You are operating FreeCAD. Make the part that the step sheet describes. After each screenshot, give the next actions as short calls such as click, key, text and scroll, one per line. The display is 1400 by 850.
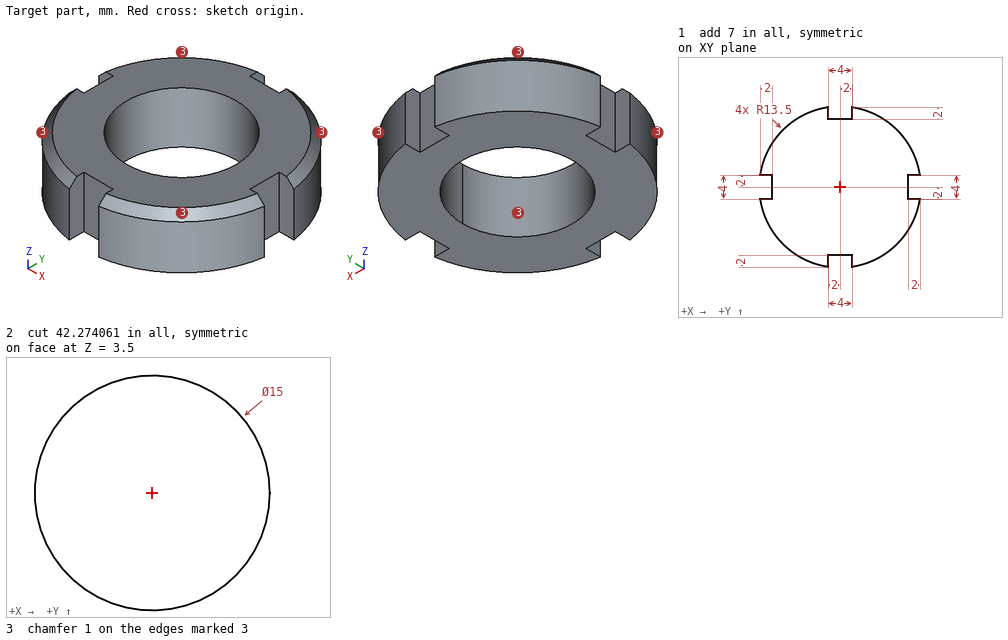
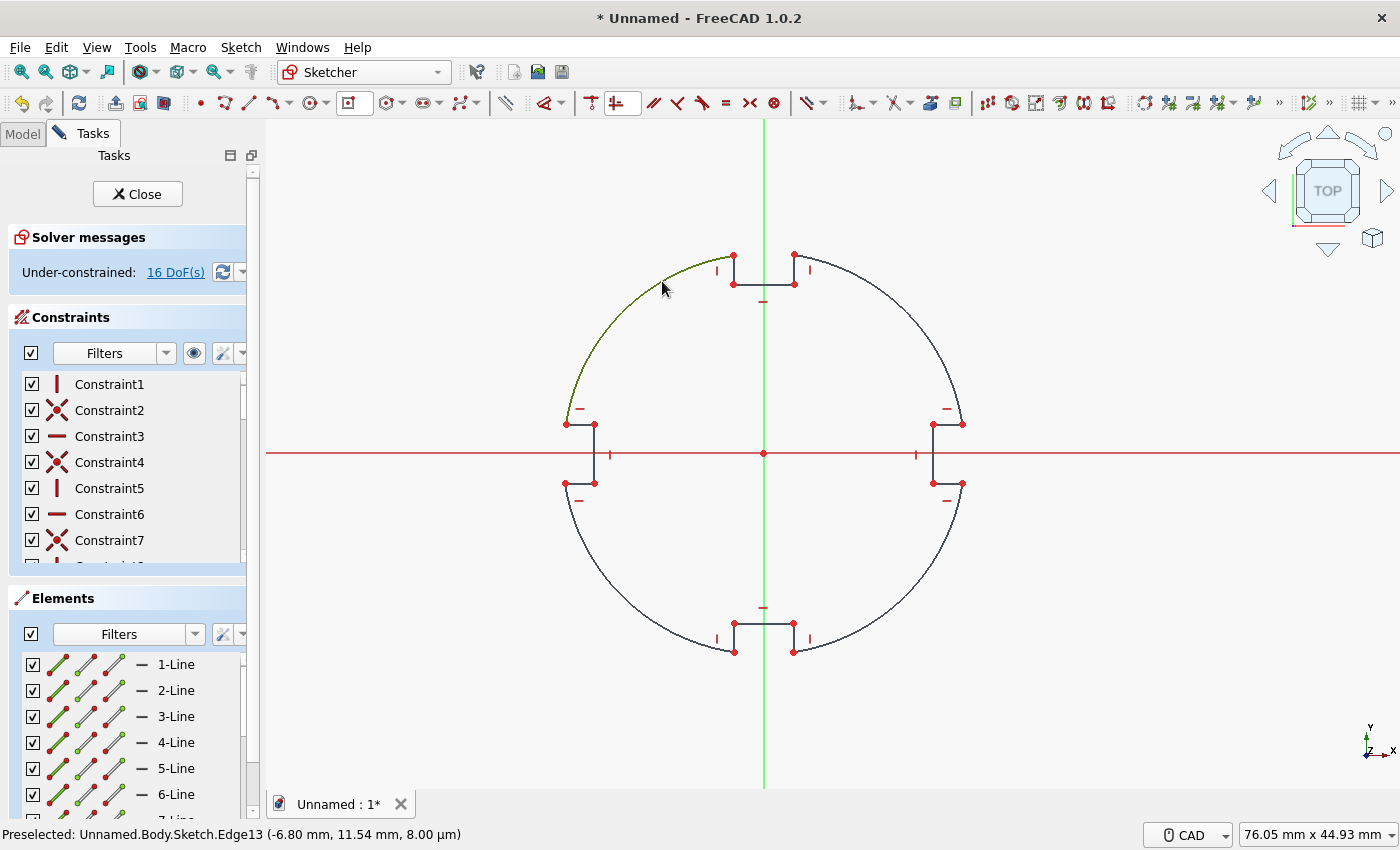
click(591, 556)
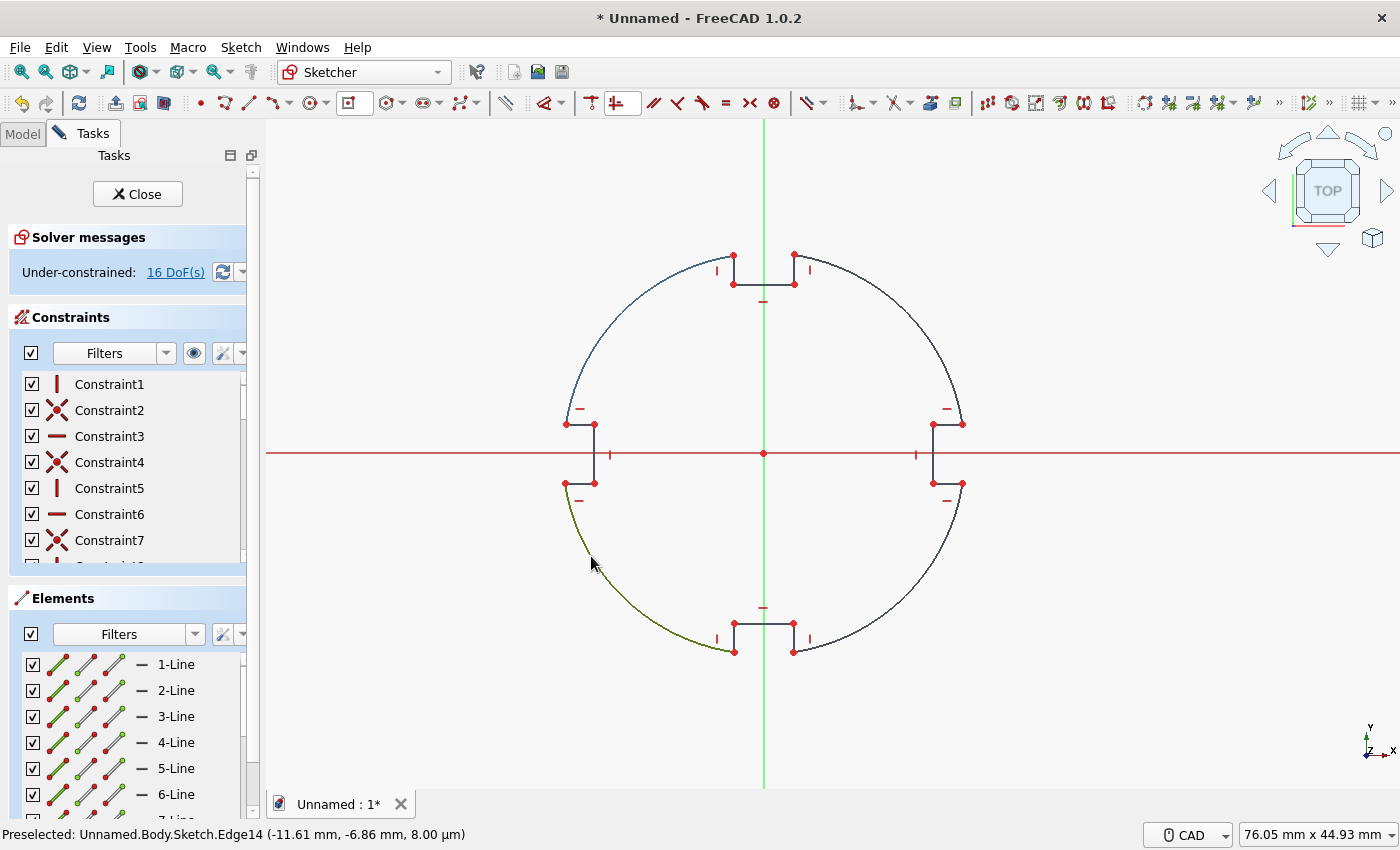
click(866, 627)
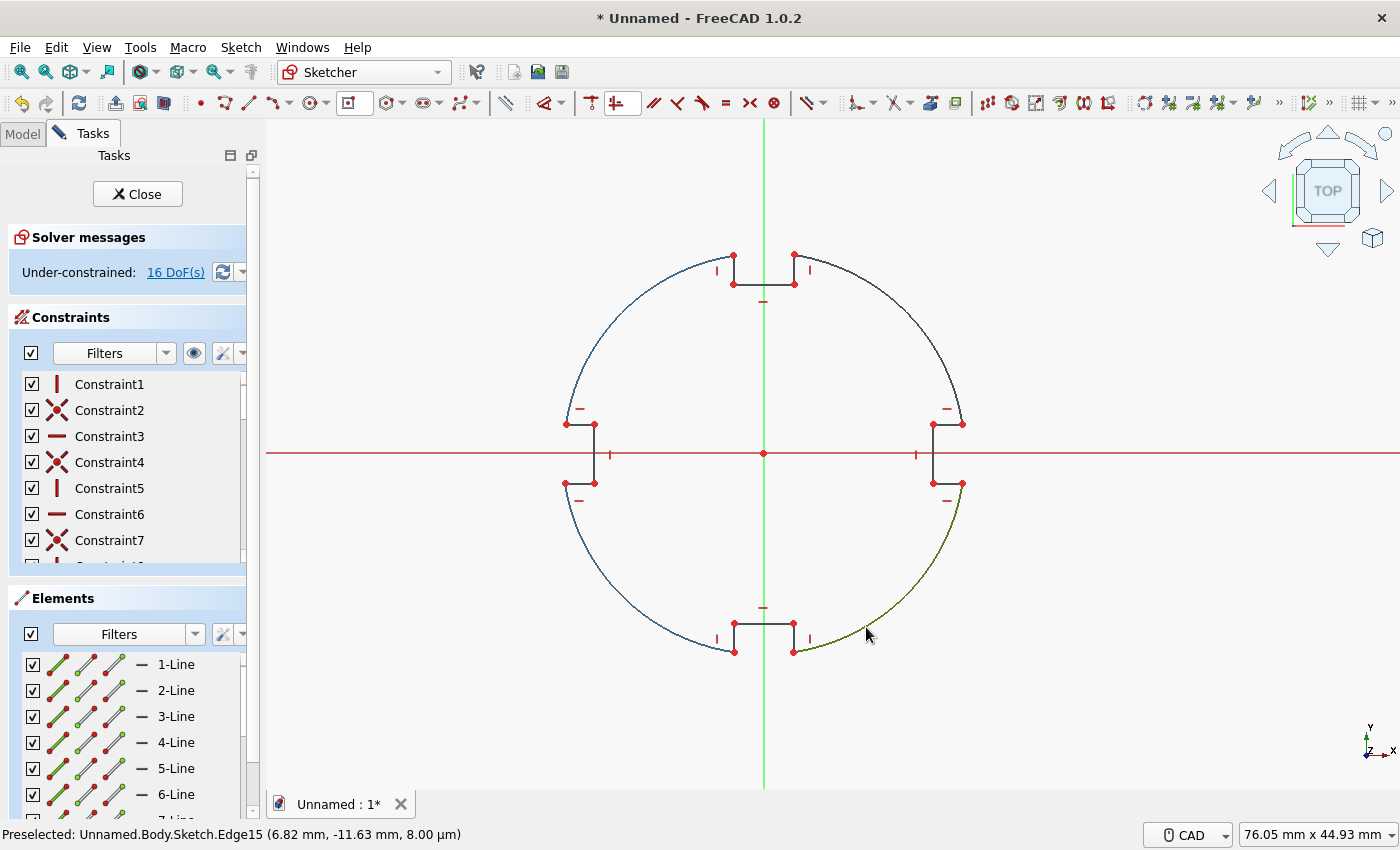
click(937, 353)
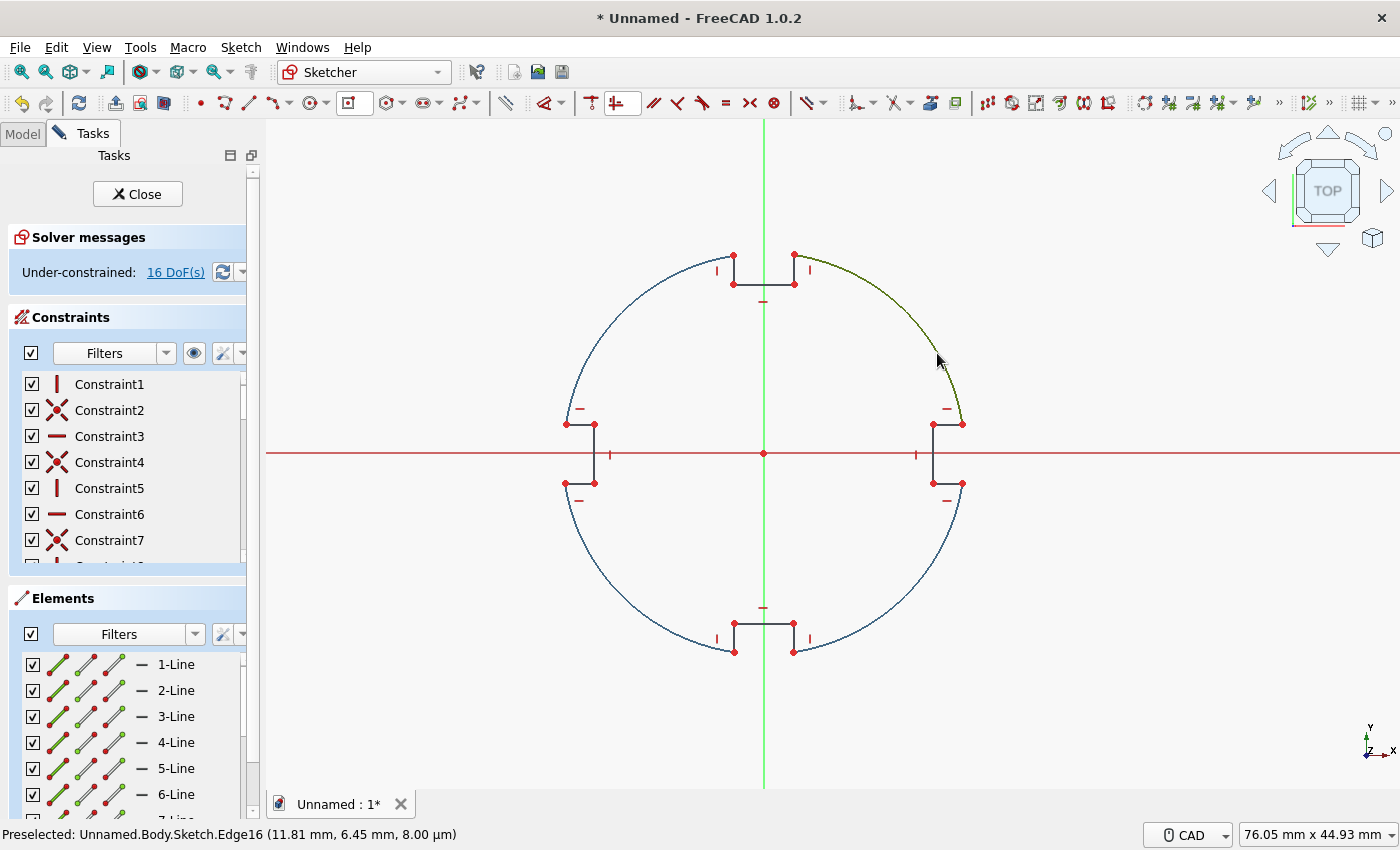
key(e)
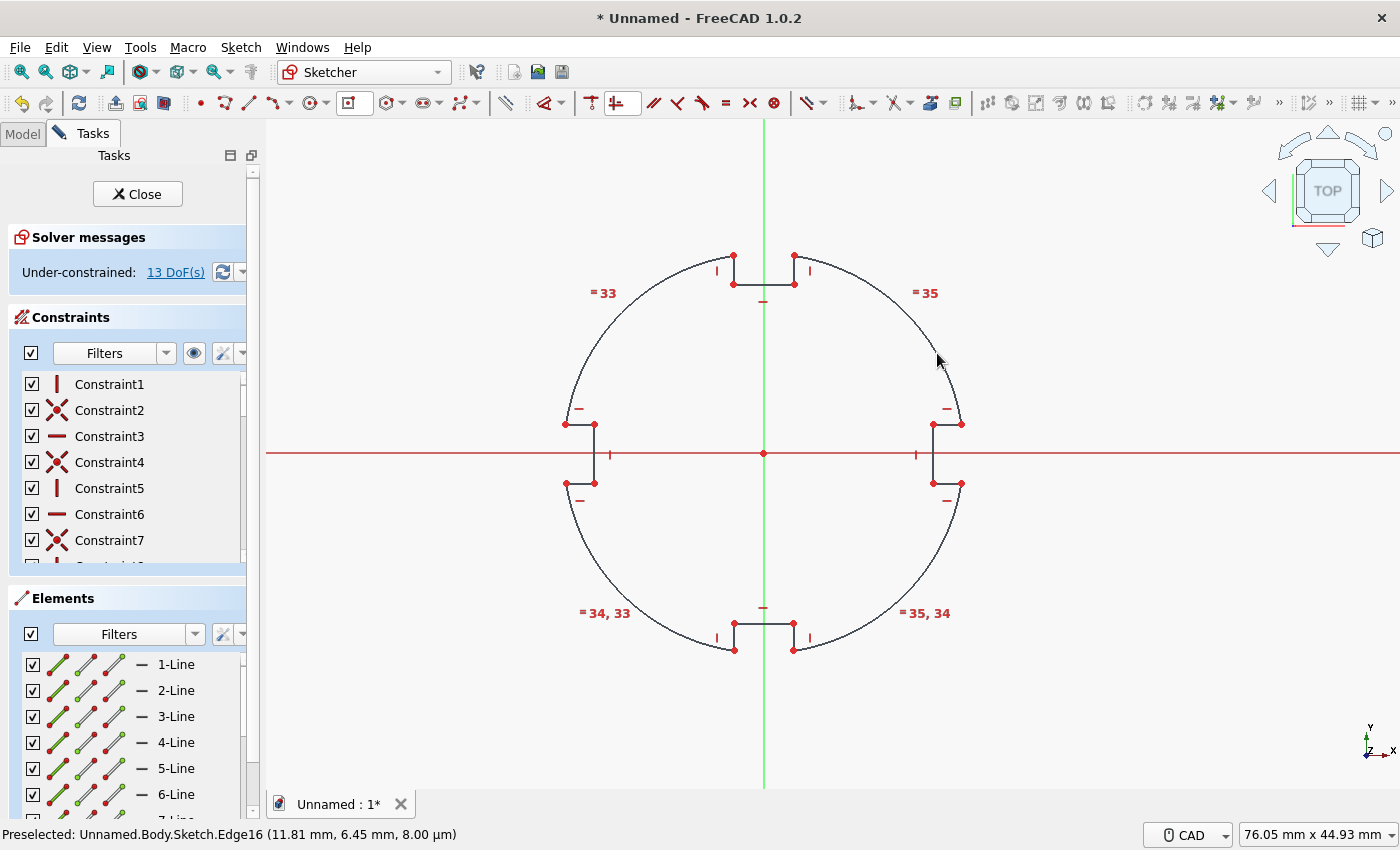
key(d)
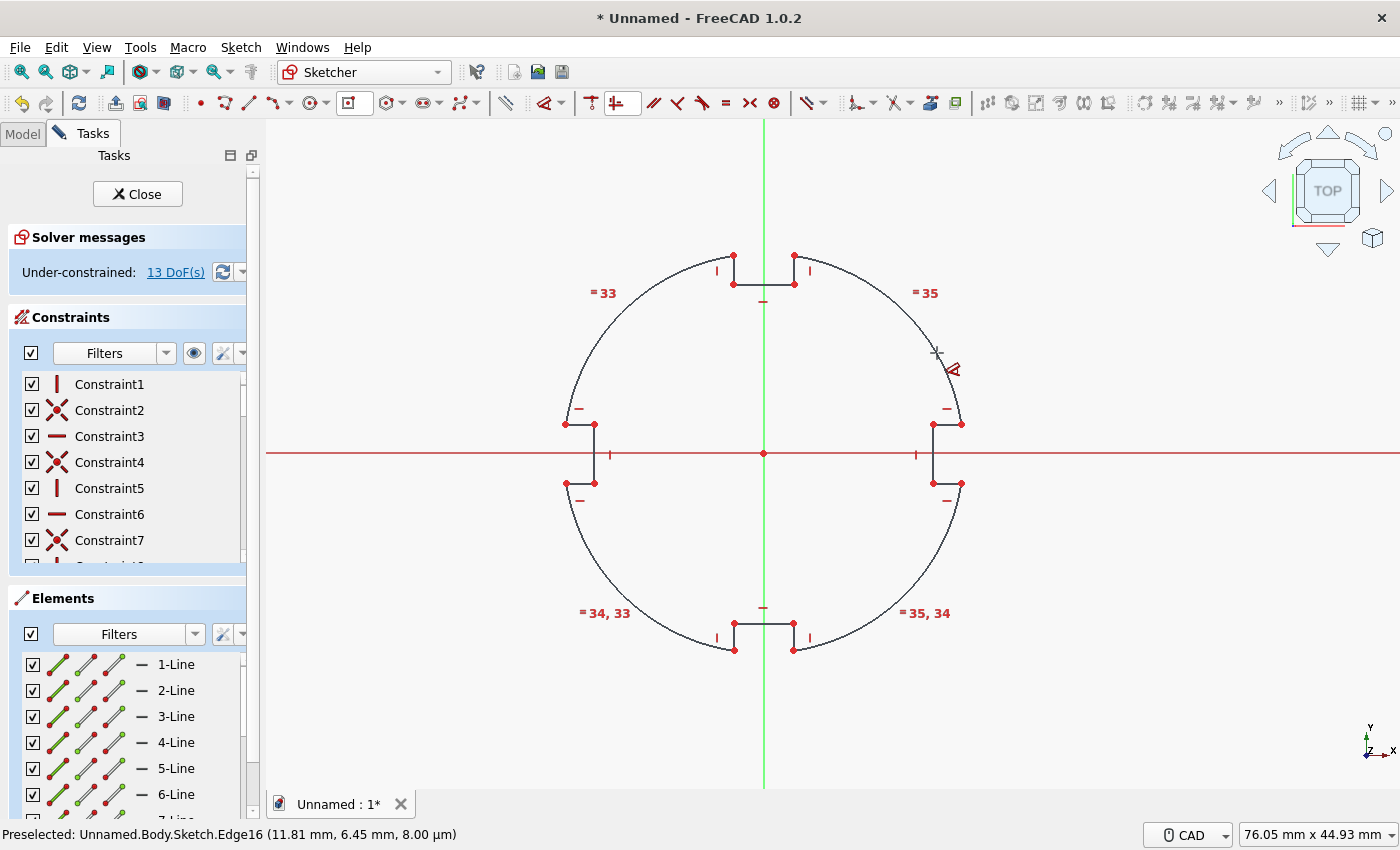
click(662, 281)
click(646, 253)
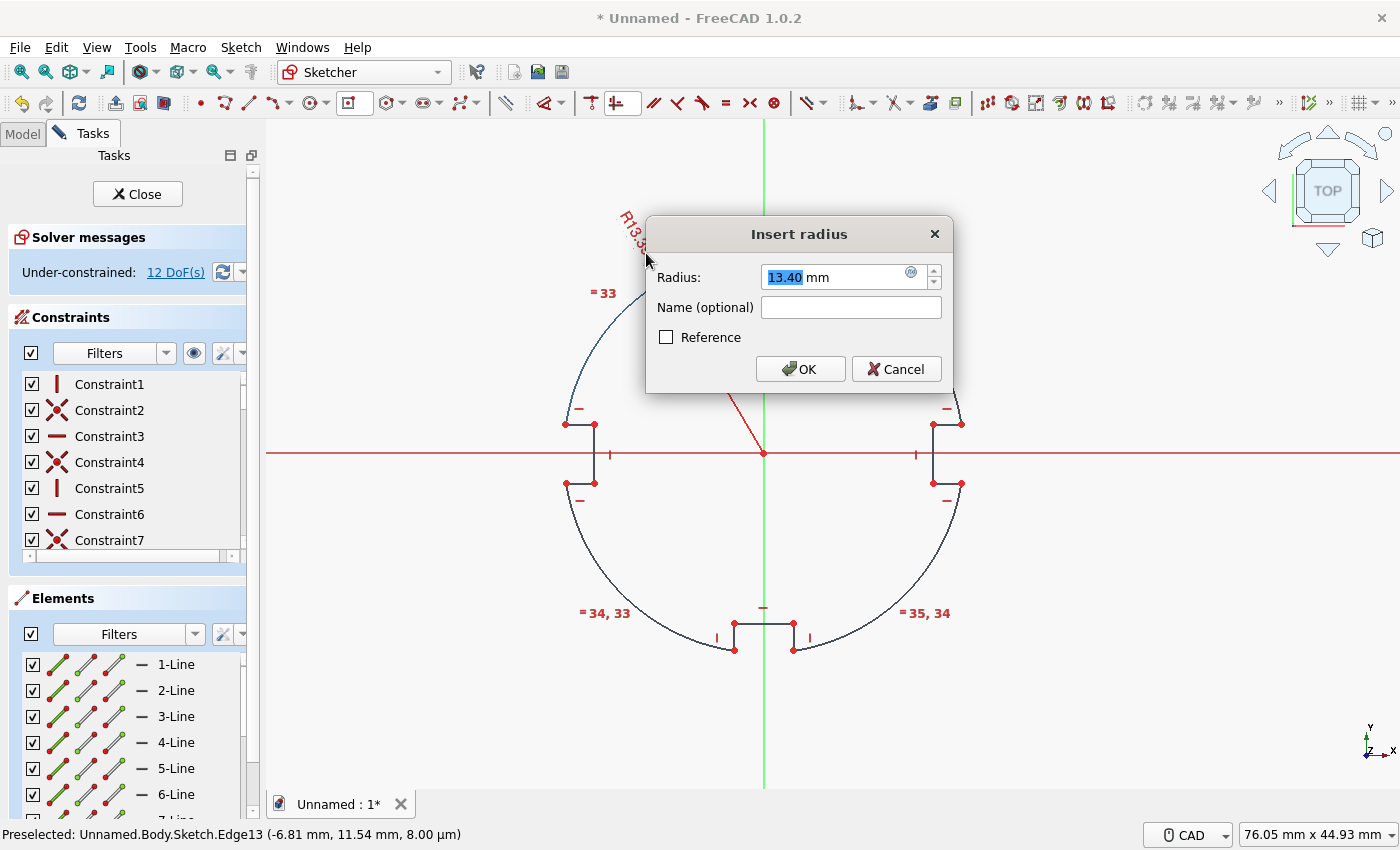
text(13.5)
key(Return)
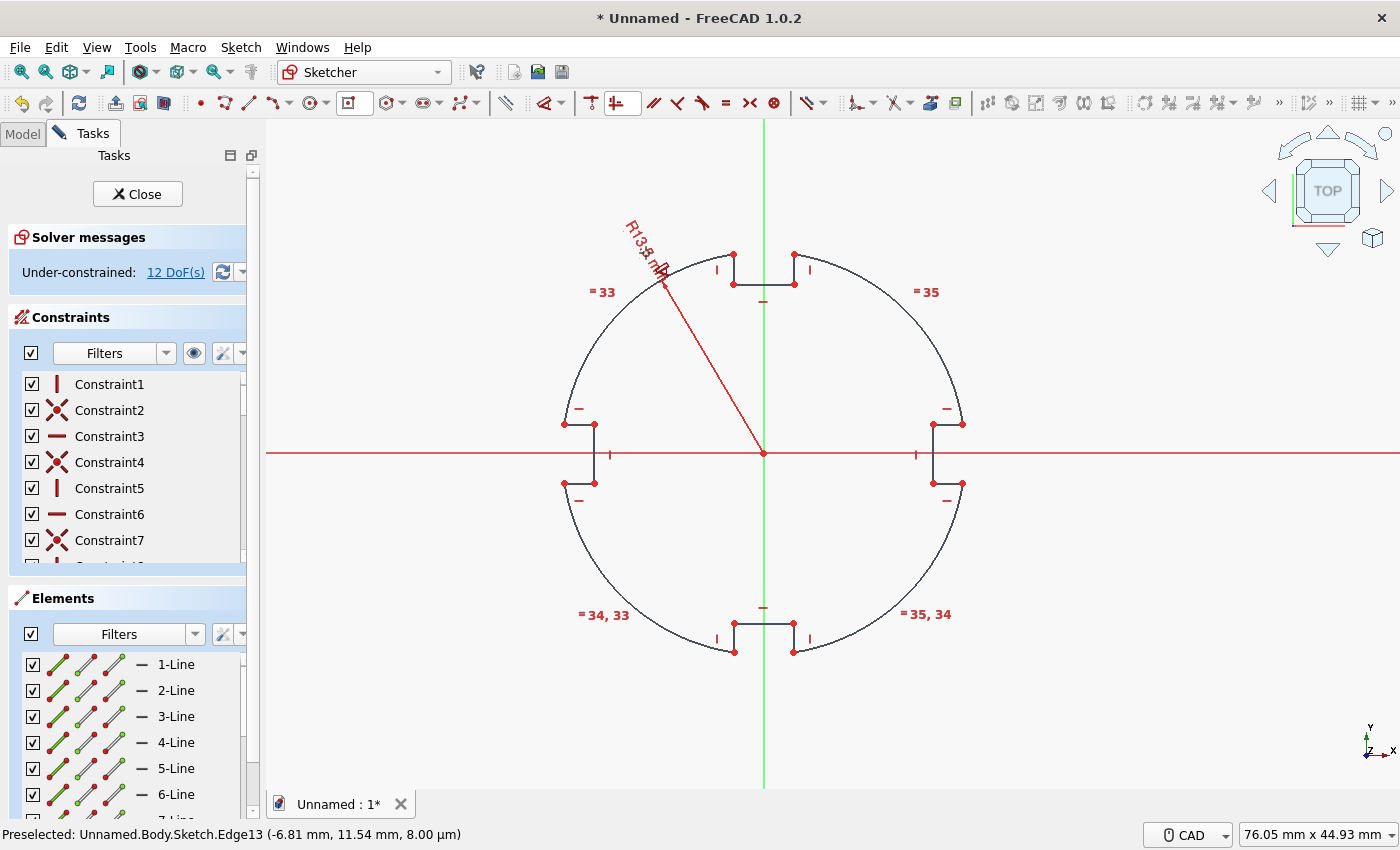
scroll(794, 264, up, 3)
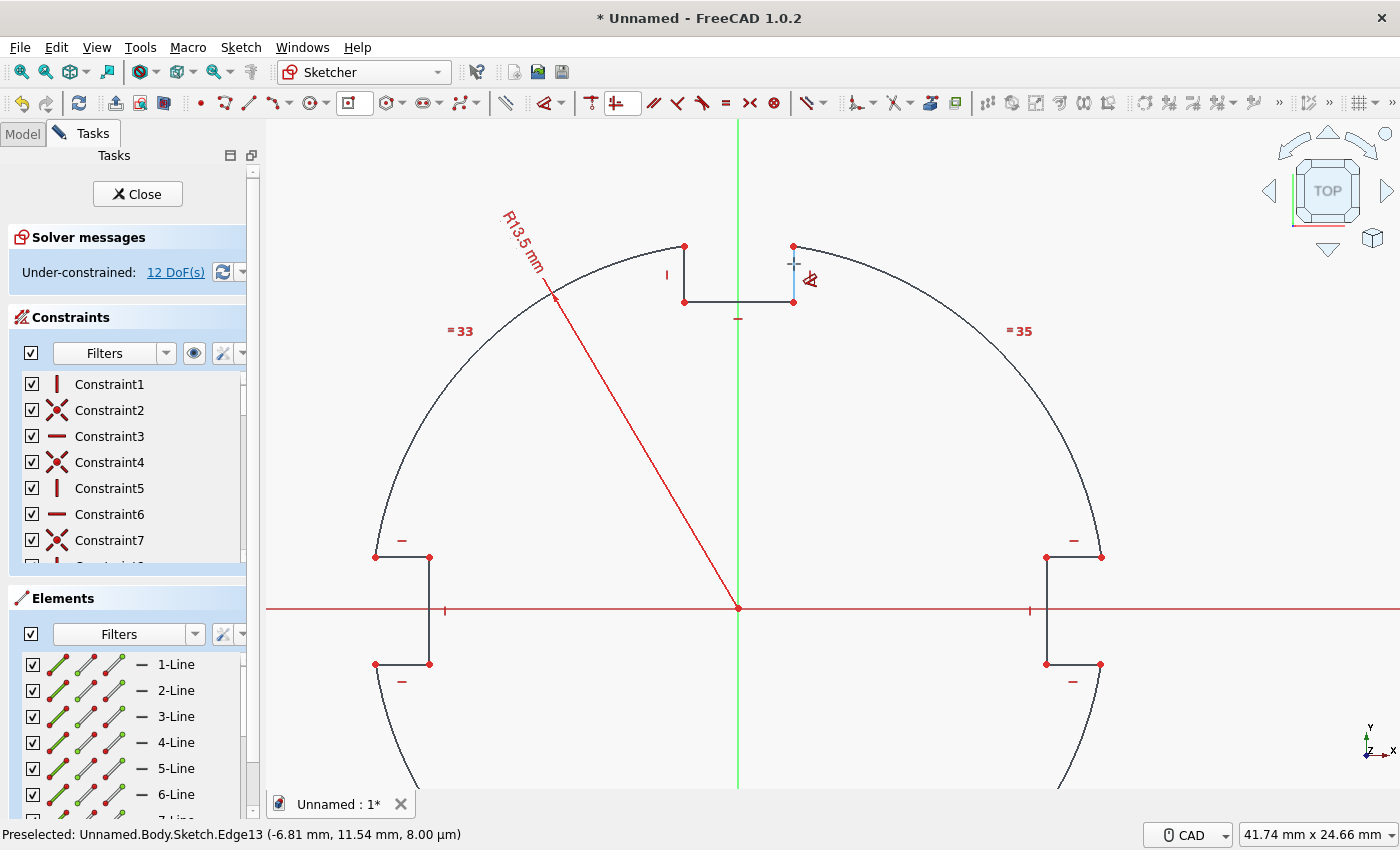
click(794, 263)
click(828, 274)